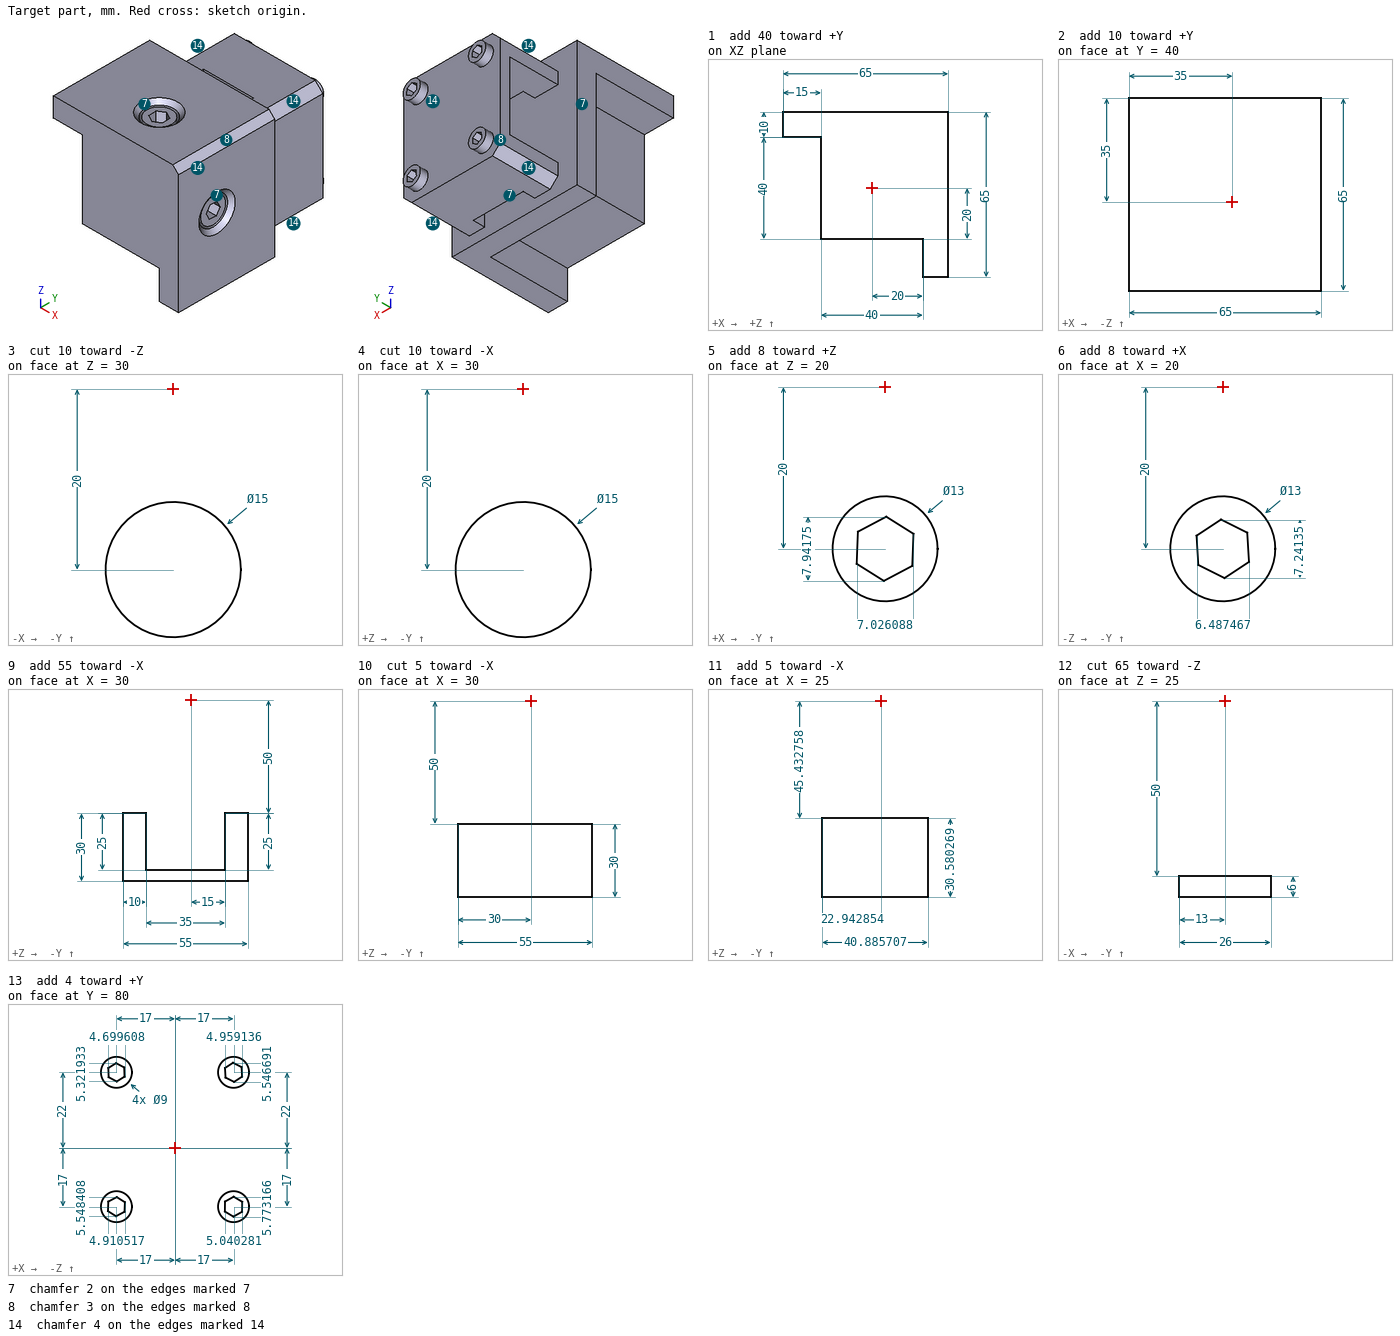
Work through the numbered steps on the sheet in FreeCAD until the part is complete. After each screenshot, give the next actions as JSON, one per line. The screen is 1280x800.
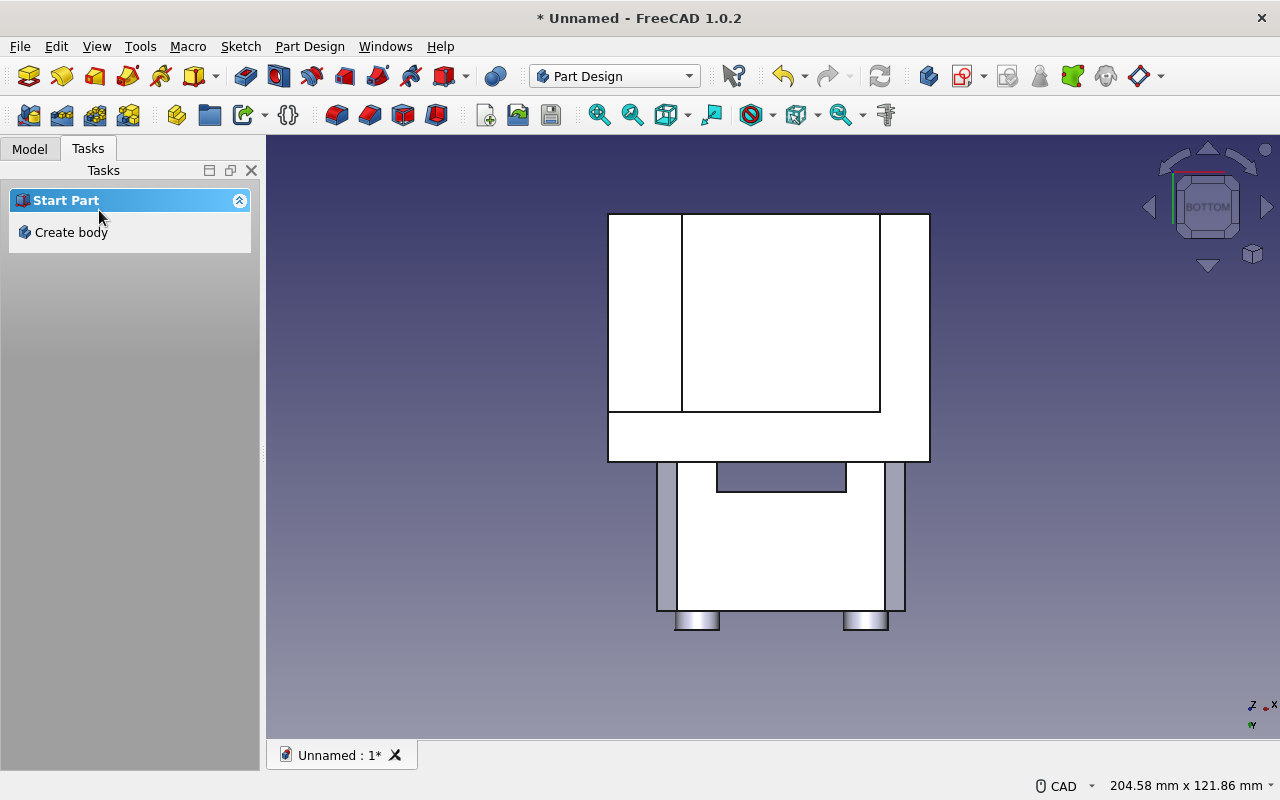
{"action": "key", "text": "0"}